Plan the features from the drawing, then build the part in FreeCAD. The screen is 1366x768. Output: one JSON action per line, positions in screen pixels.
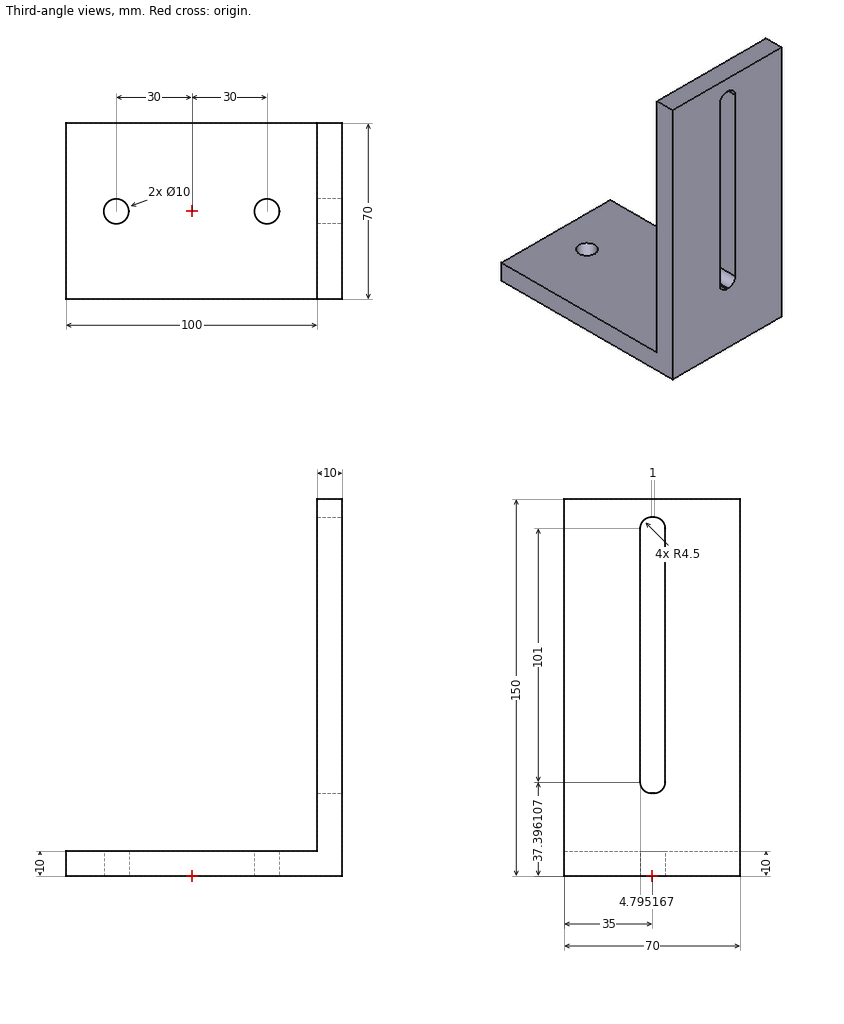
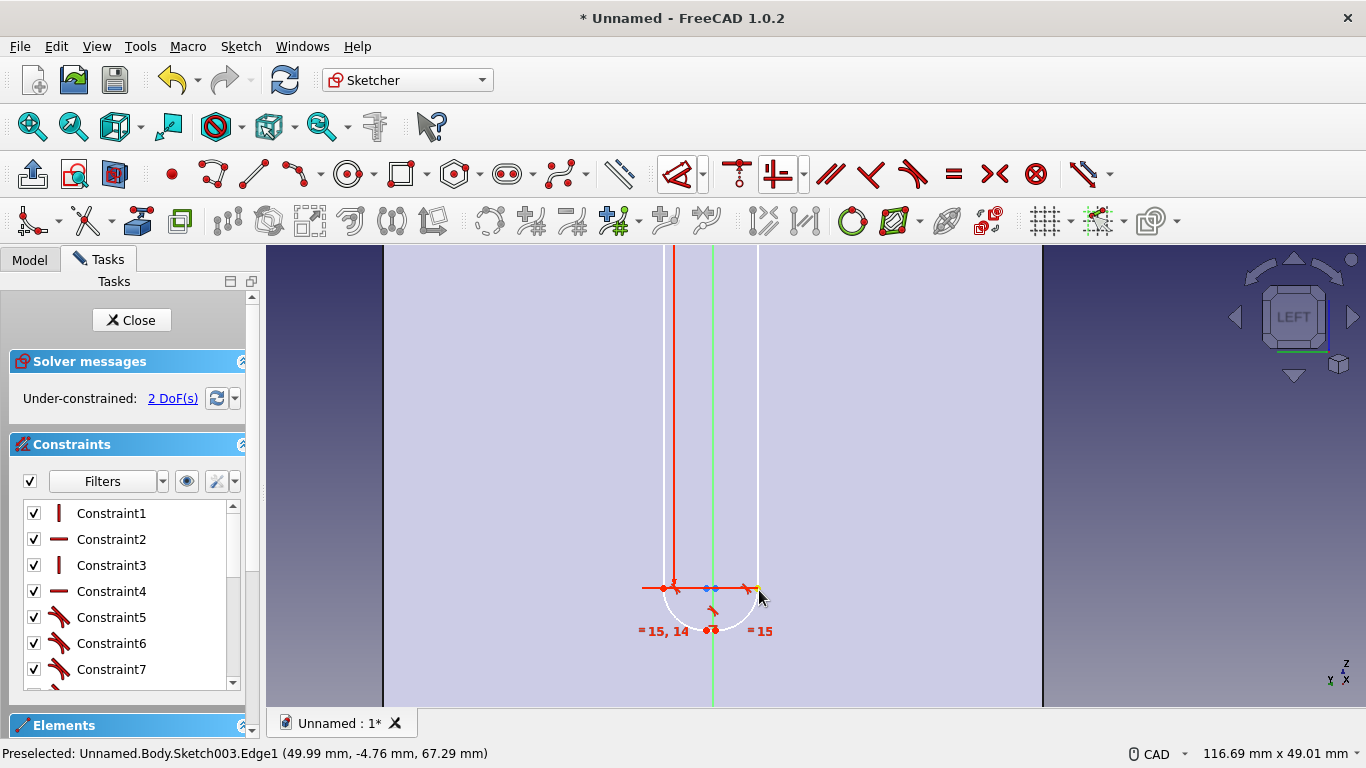
{"action": "left_click", "coordinate": [758, 588]}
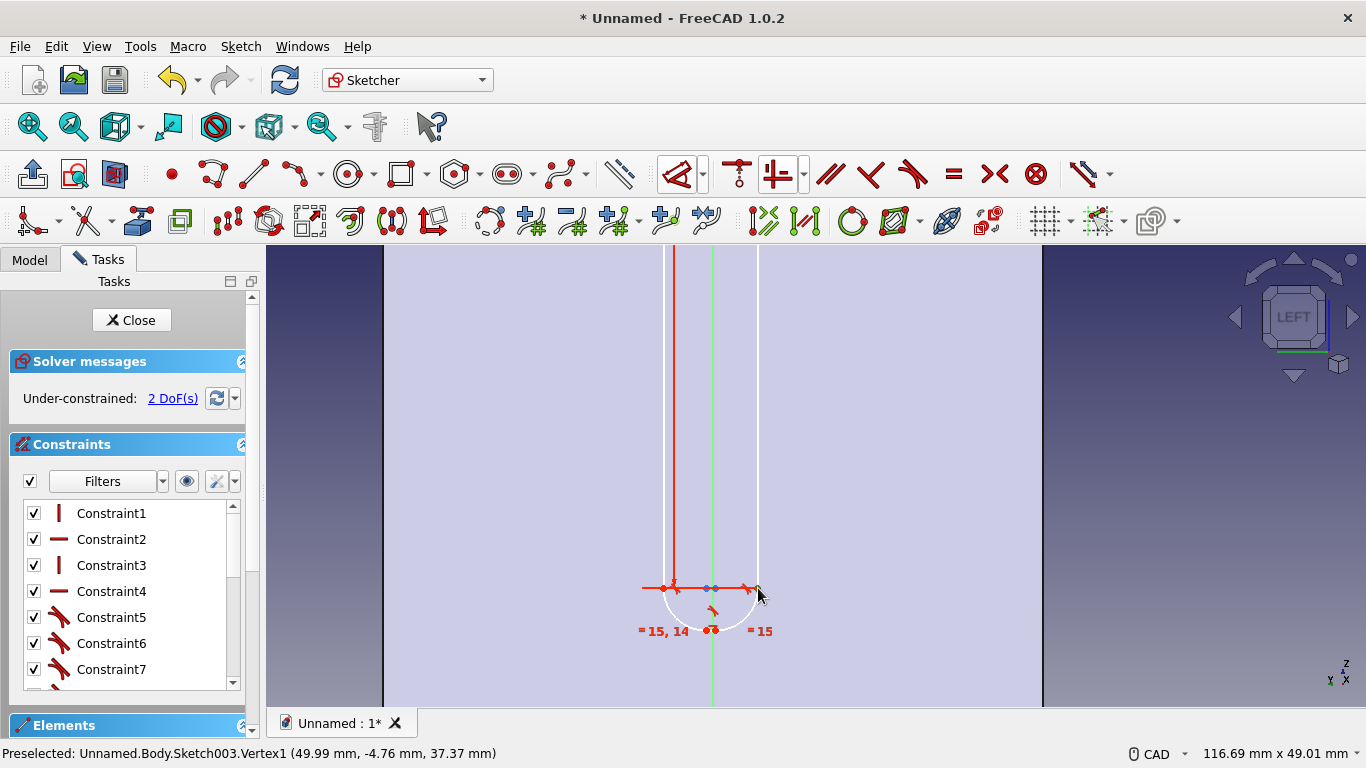
{"action": "left_click", "coordinate": [702, 174]}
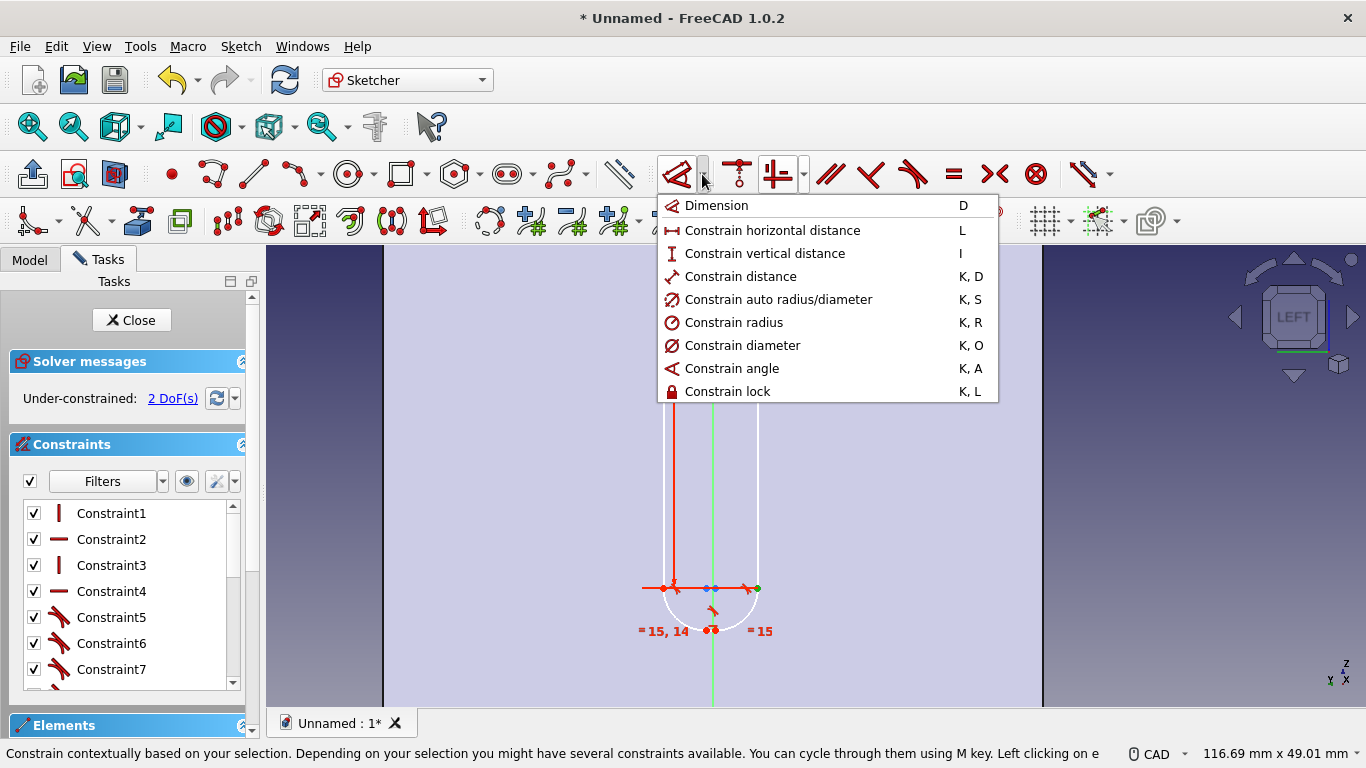
{"action": "left_click", "coordinate": [828, 230]}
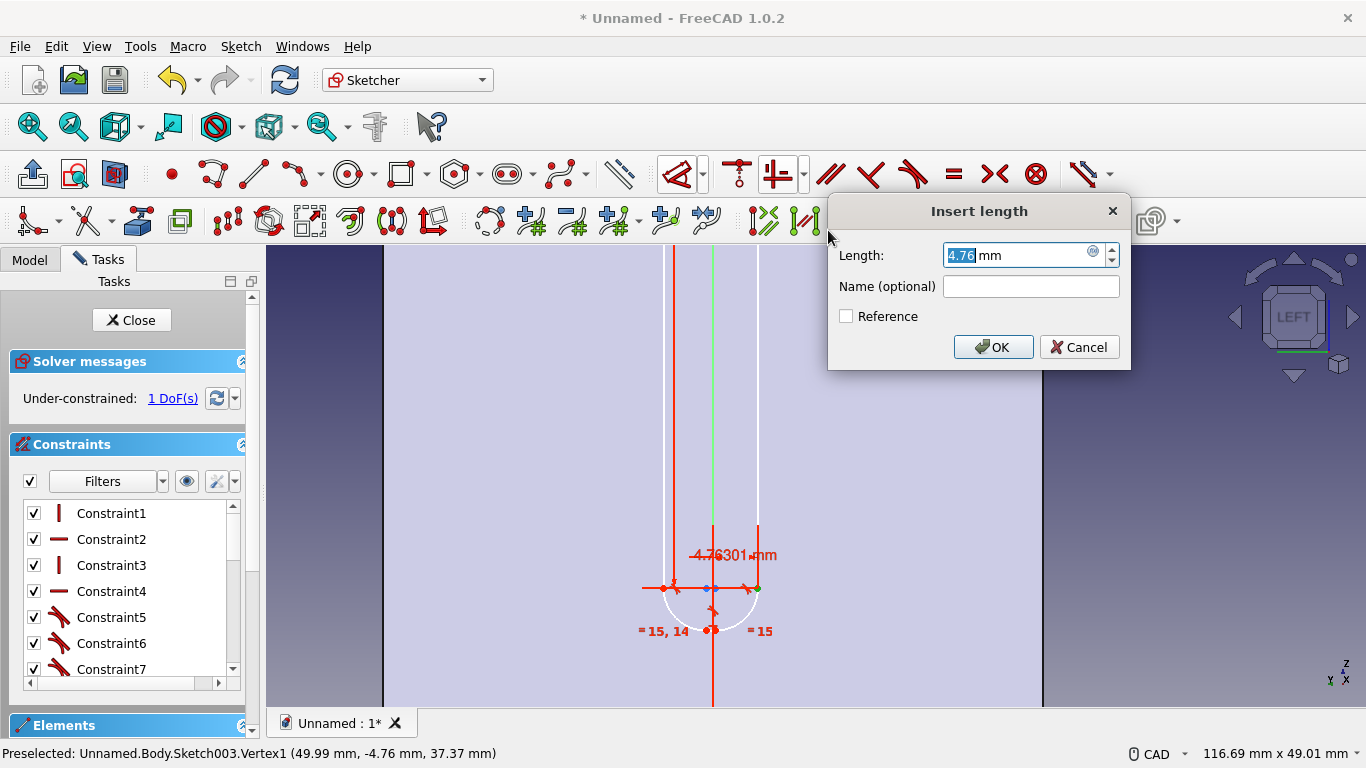
{"action": "type", "text": "4.795167"}
{"action": "key", "text": "Return"}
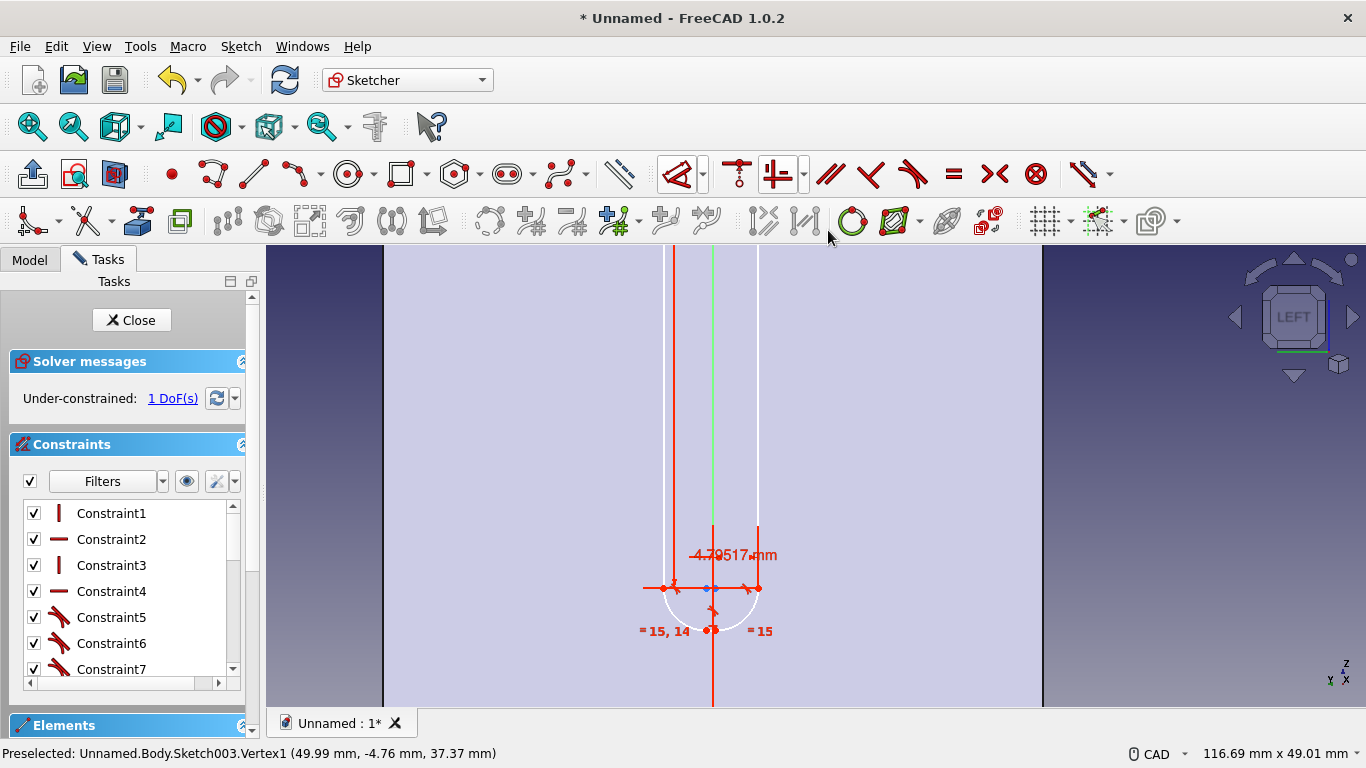
{"action": "scroll", "coordinate": [757, 529], "scroll_direction": "down", "scroll_amount": 8}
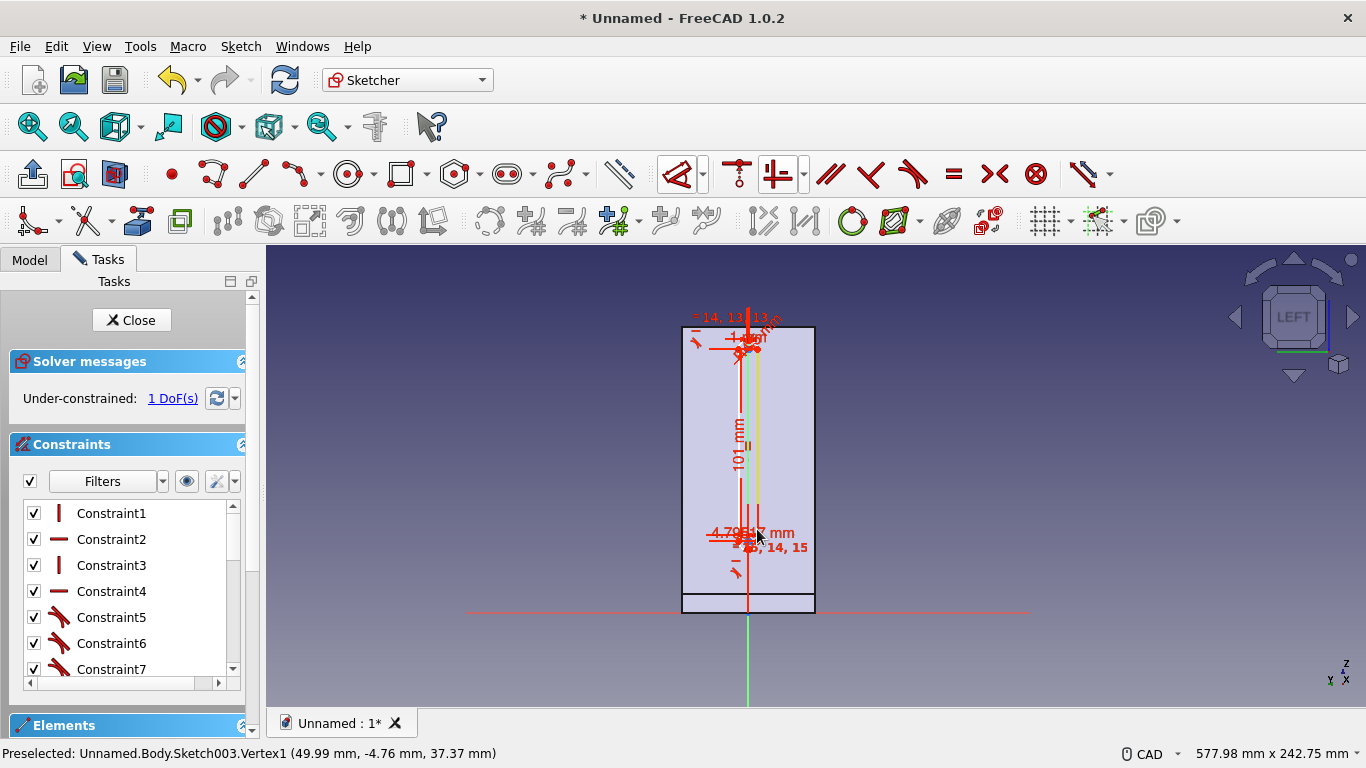
{"action": "scroll", "coordinate": [758, 541], "scroll_direction": "up", "scroll_amount": 2}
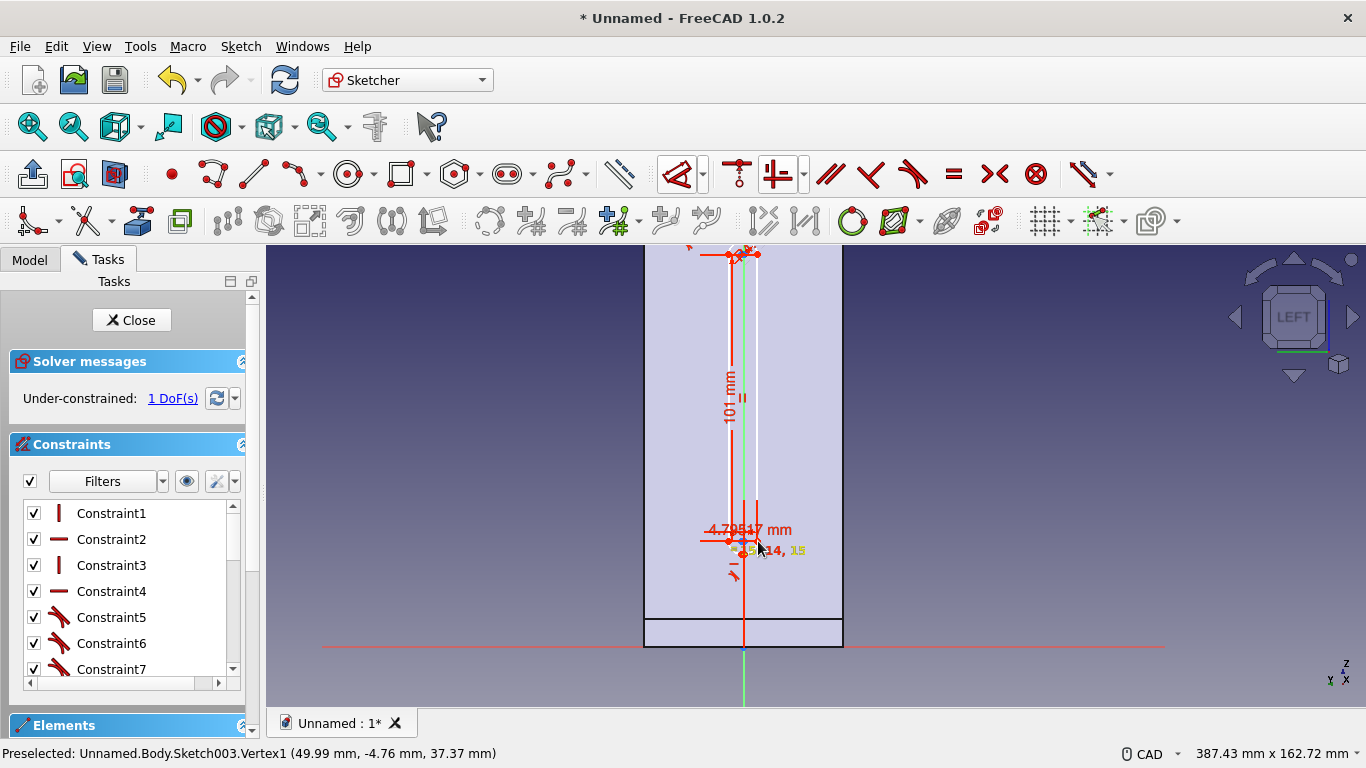
{"action": "left_click", "coordinate": [757, 541]}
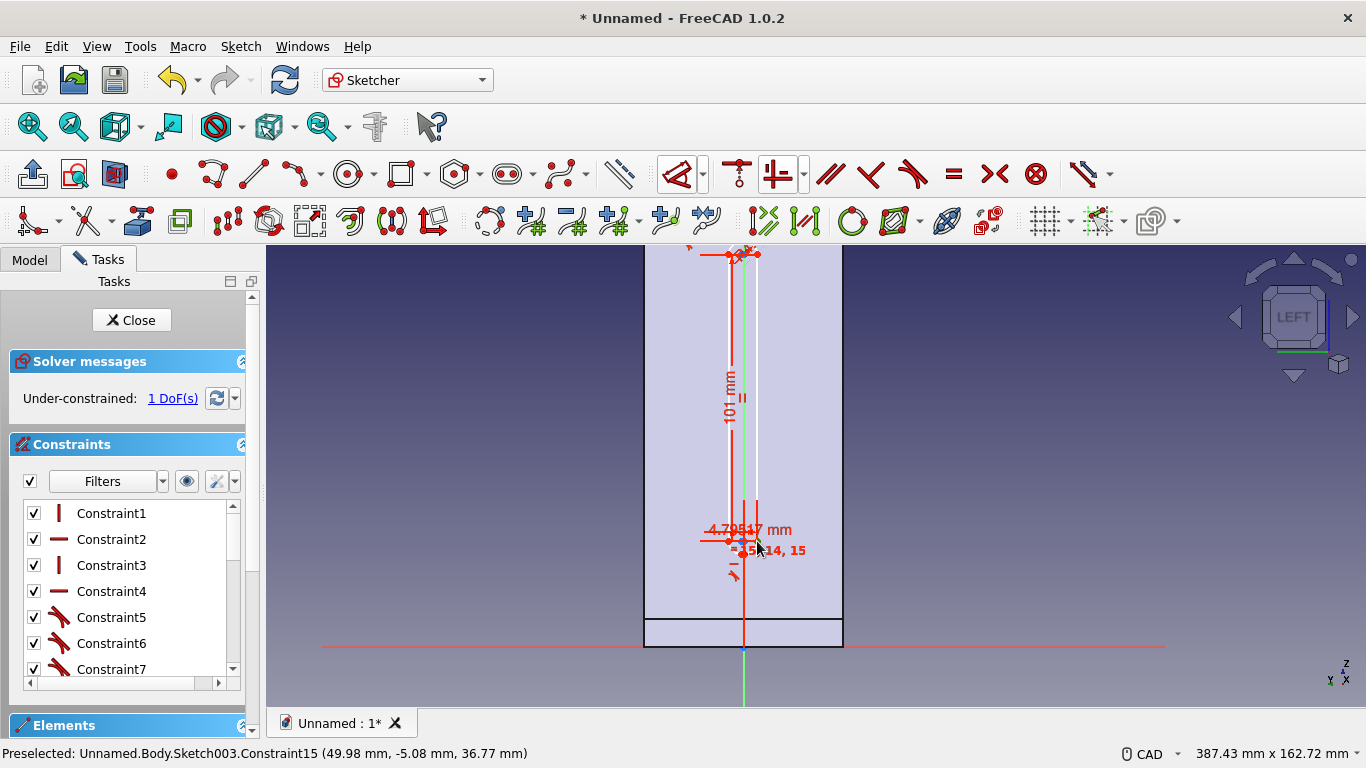
{"action": "key", "text": "i"}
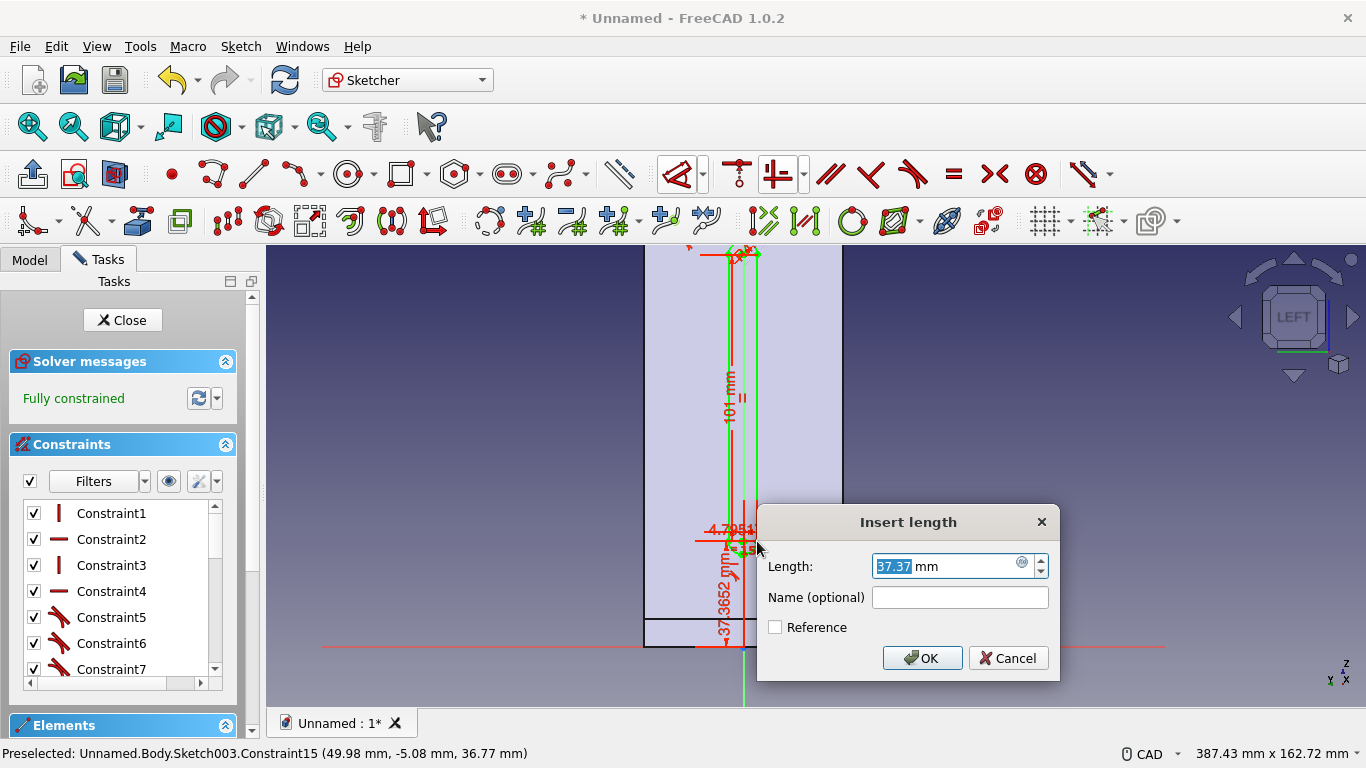
{"action": "type", "text": "37.396107"}
{"action": "key", "text": "Return"}